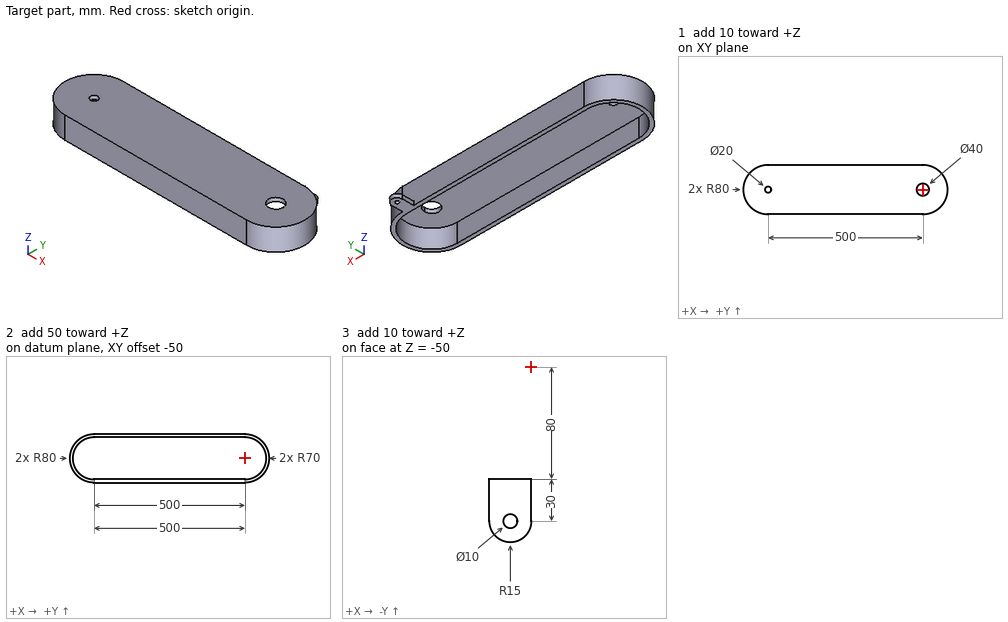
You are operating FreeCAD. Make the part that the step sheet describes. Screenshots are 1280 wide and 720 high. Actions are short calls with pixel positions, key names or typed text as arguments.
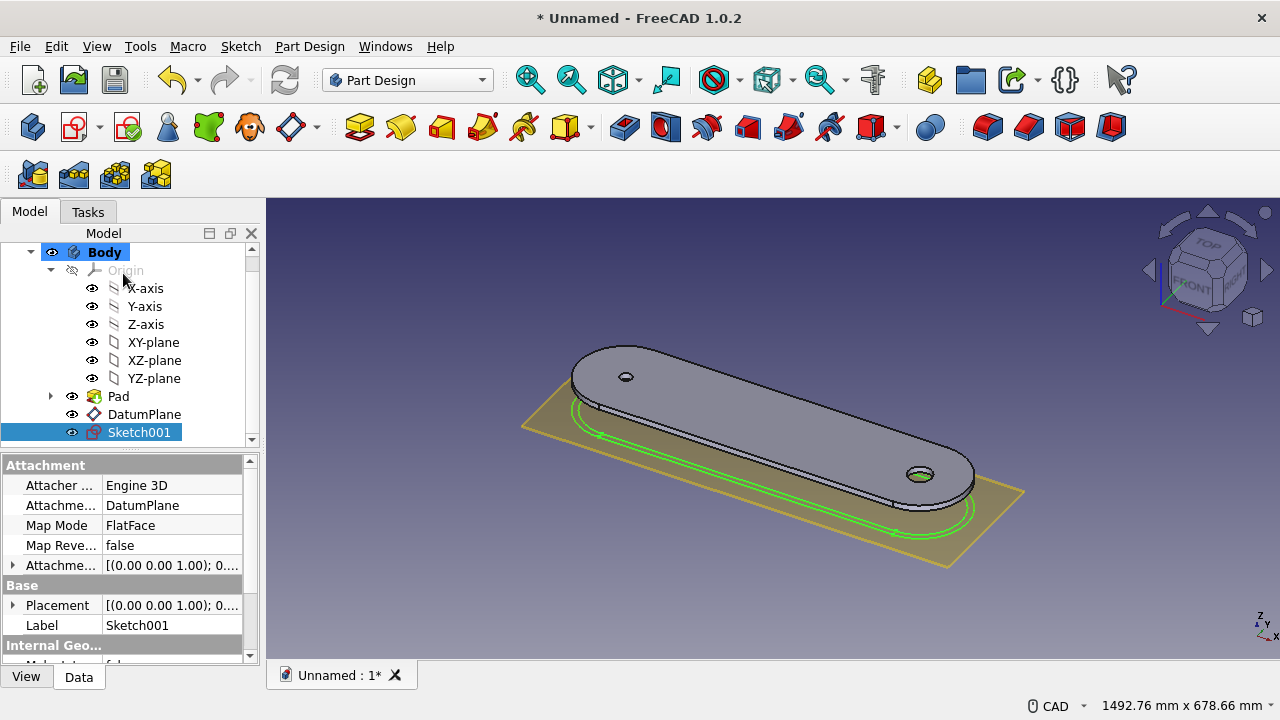
click(360, 128)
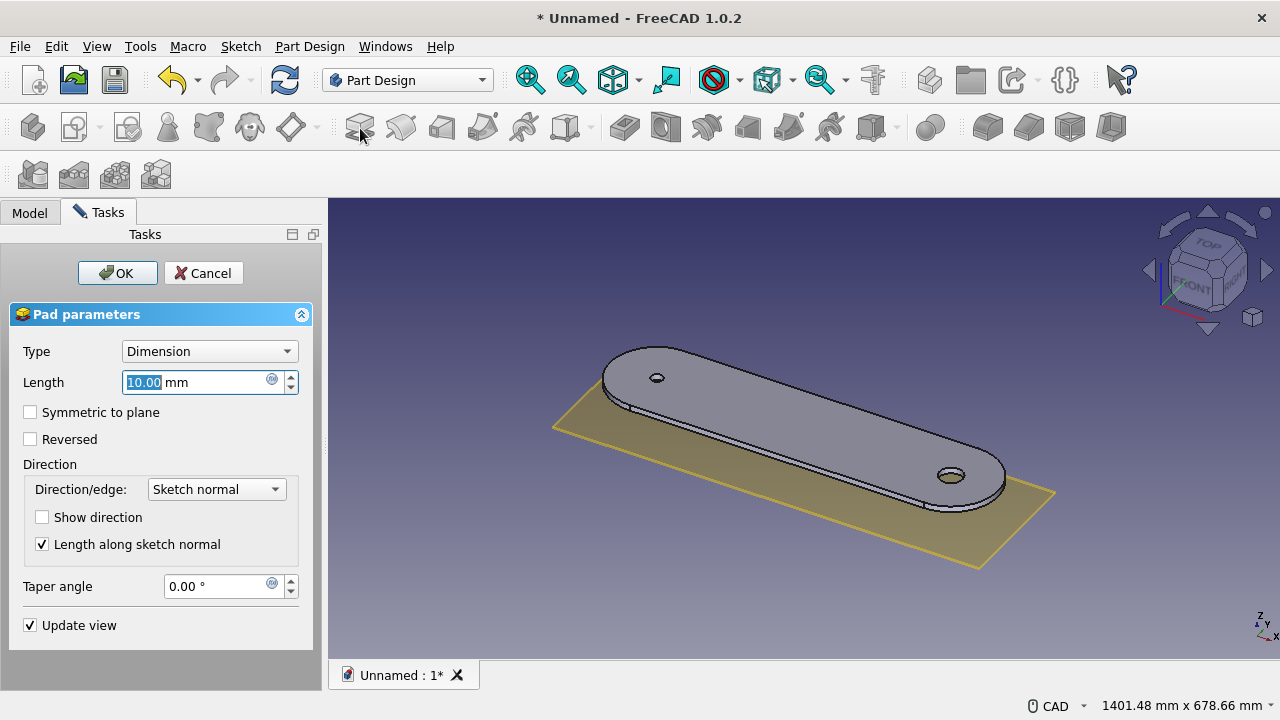
text(50)
key(Tab)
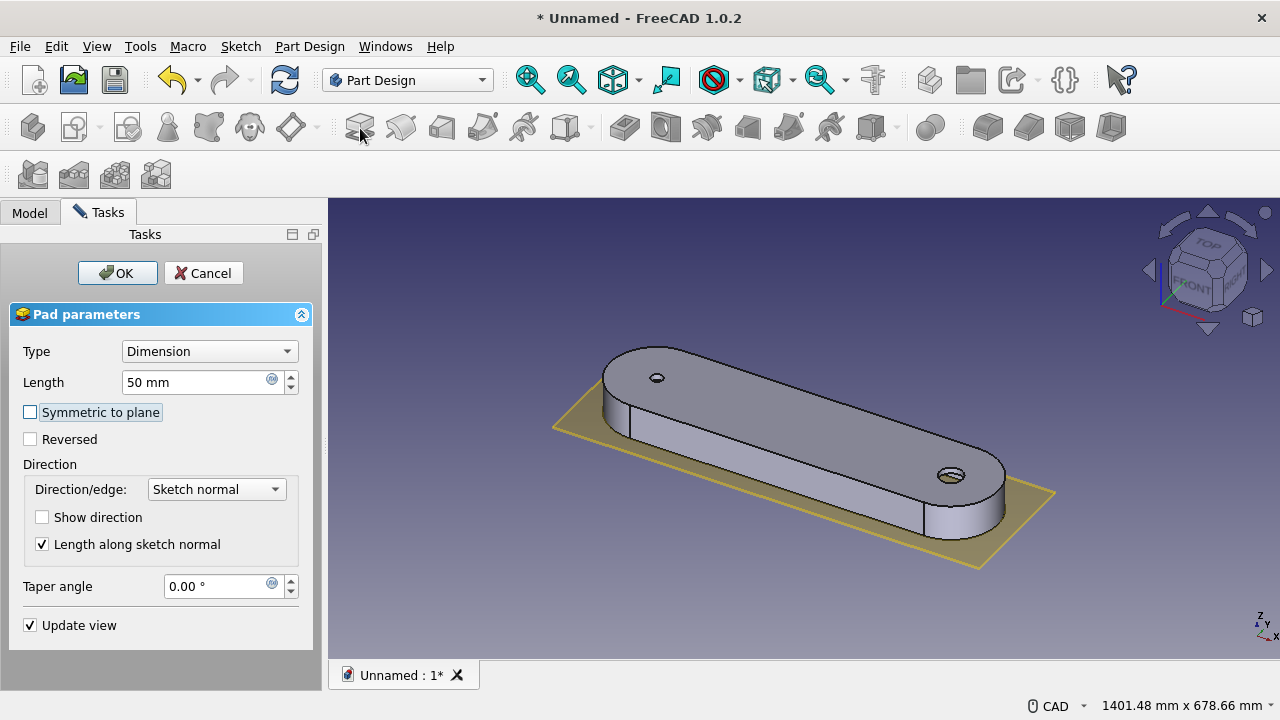
click(118, 273)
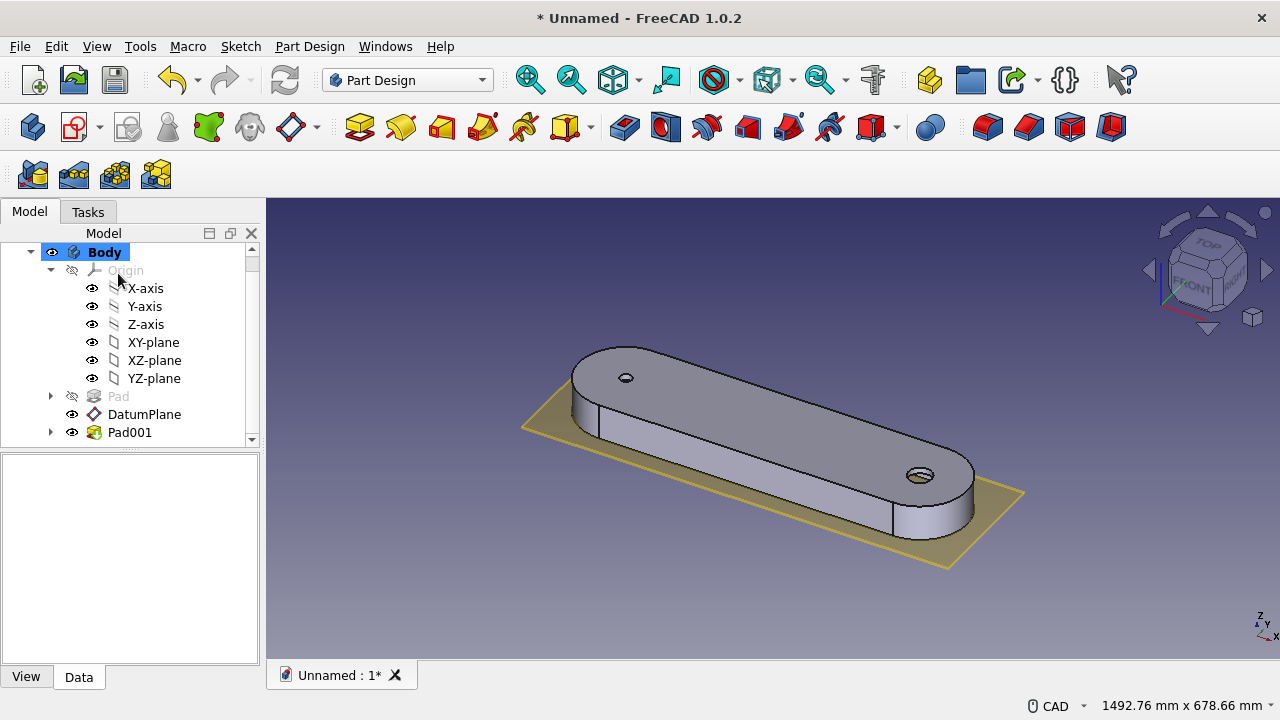
click(117, 414)
key(space)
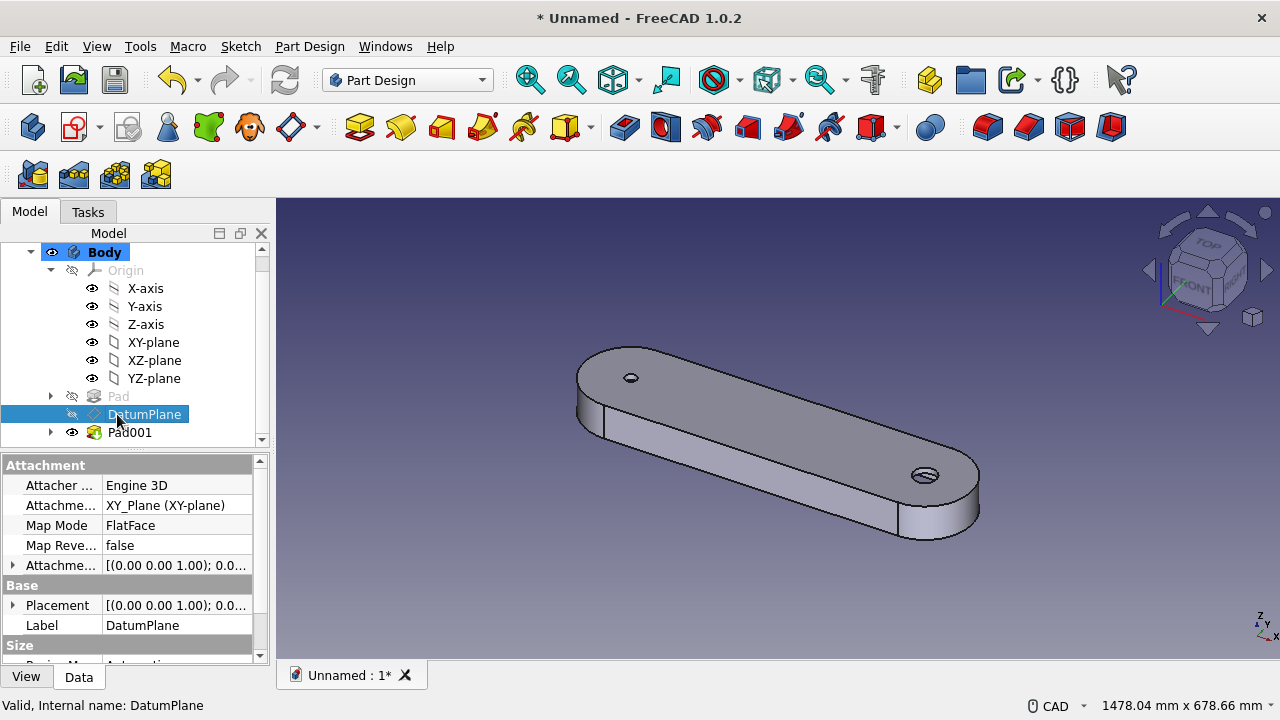
key(5)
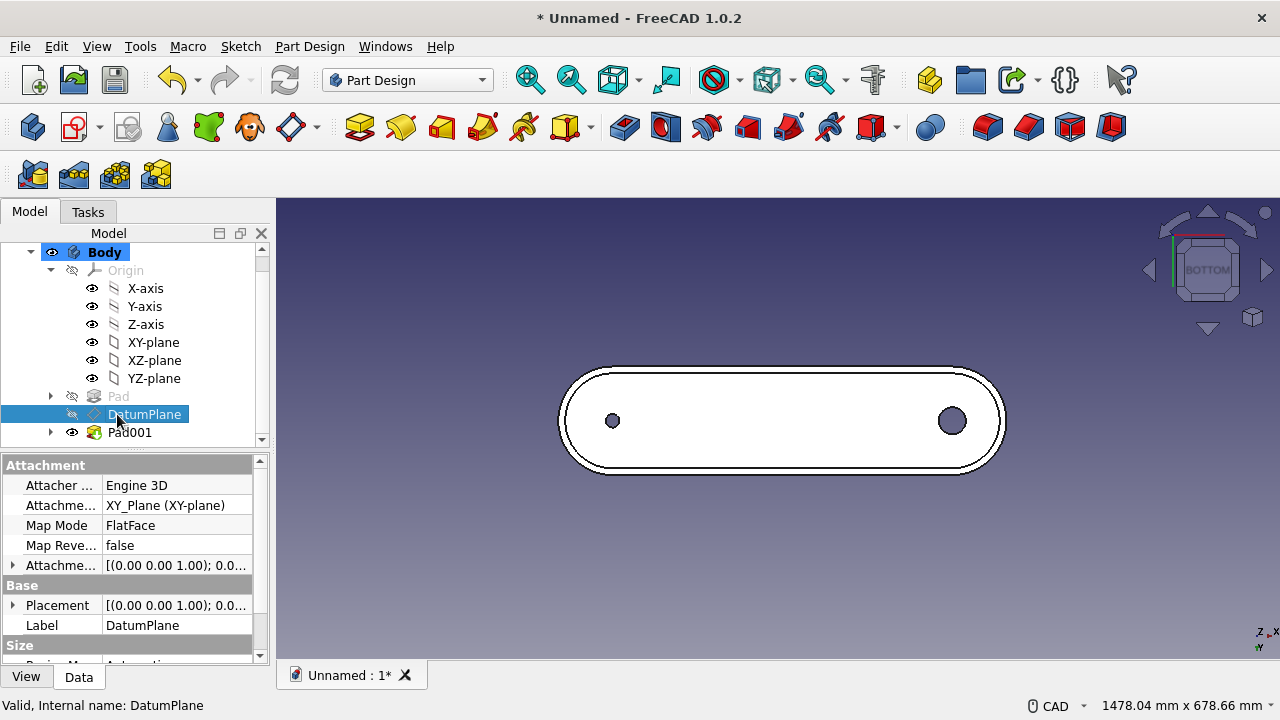
click(531, 80)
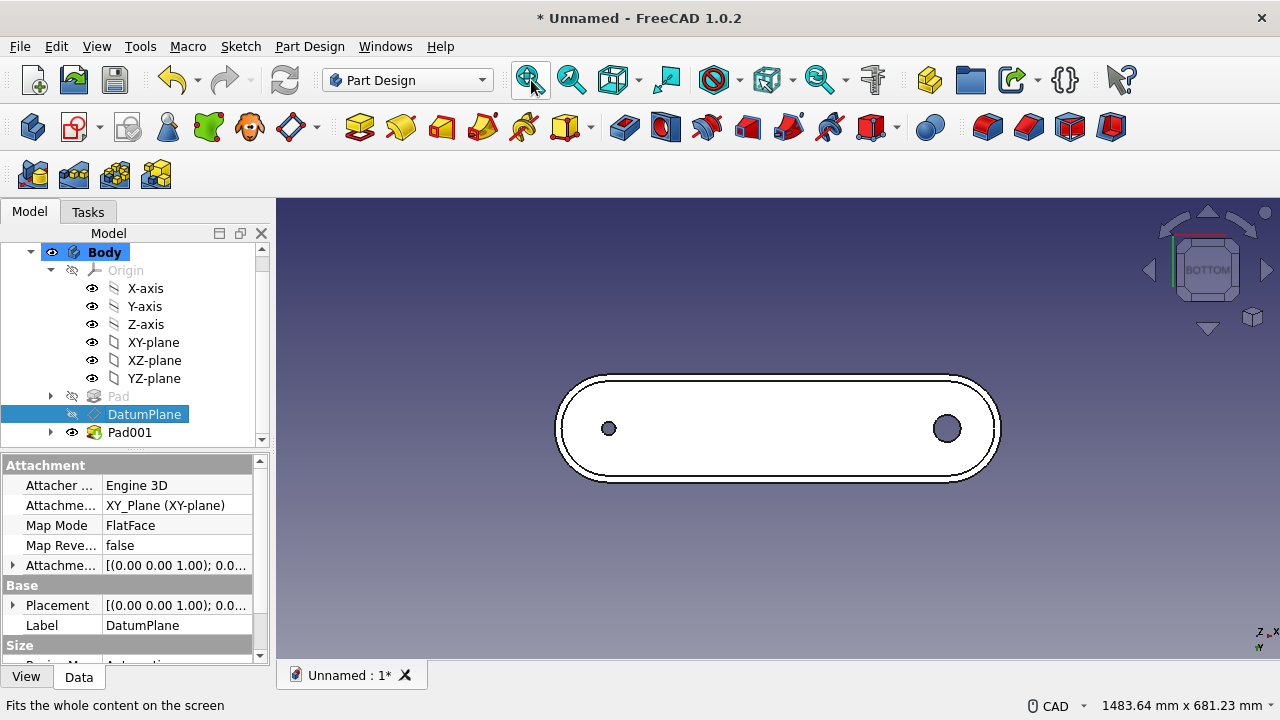
scroll(969, 381, up, 8)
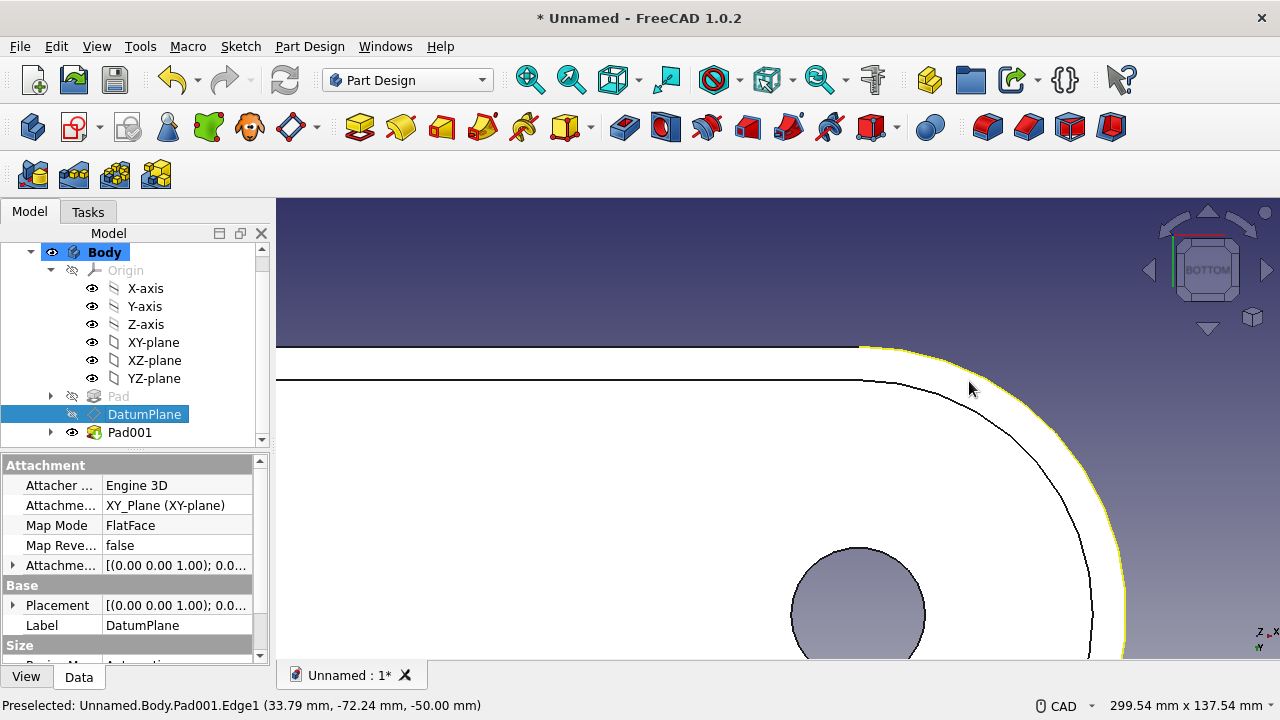
click(968, 384)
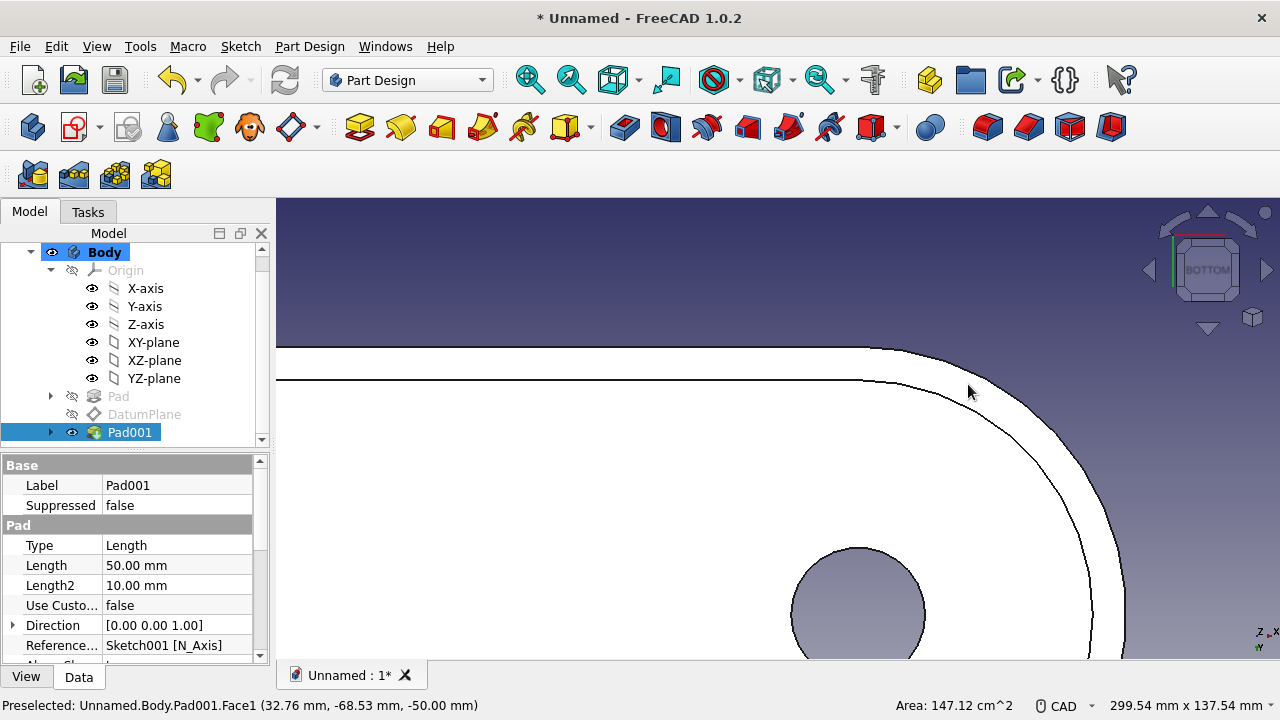
click(74, 128)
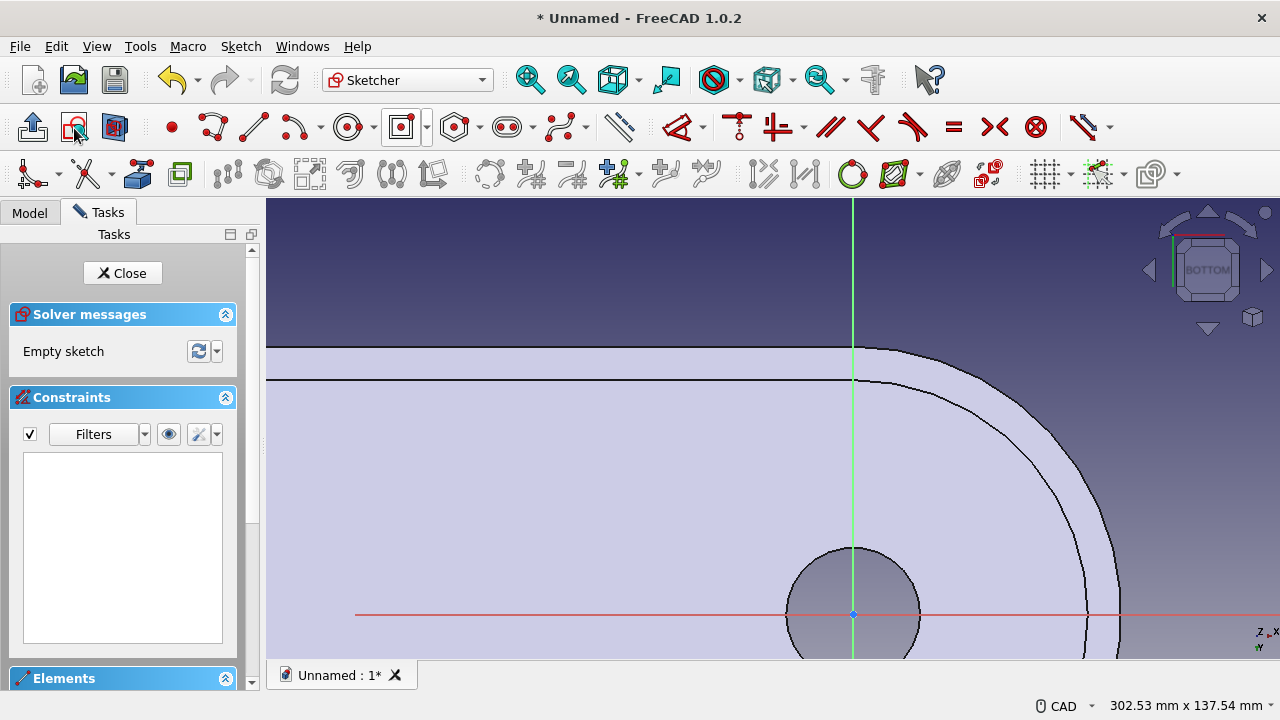
scroll(704, 428, down, 5)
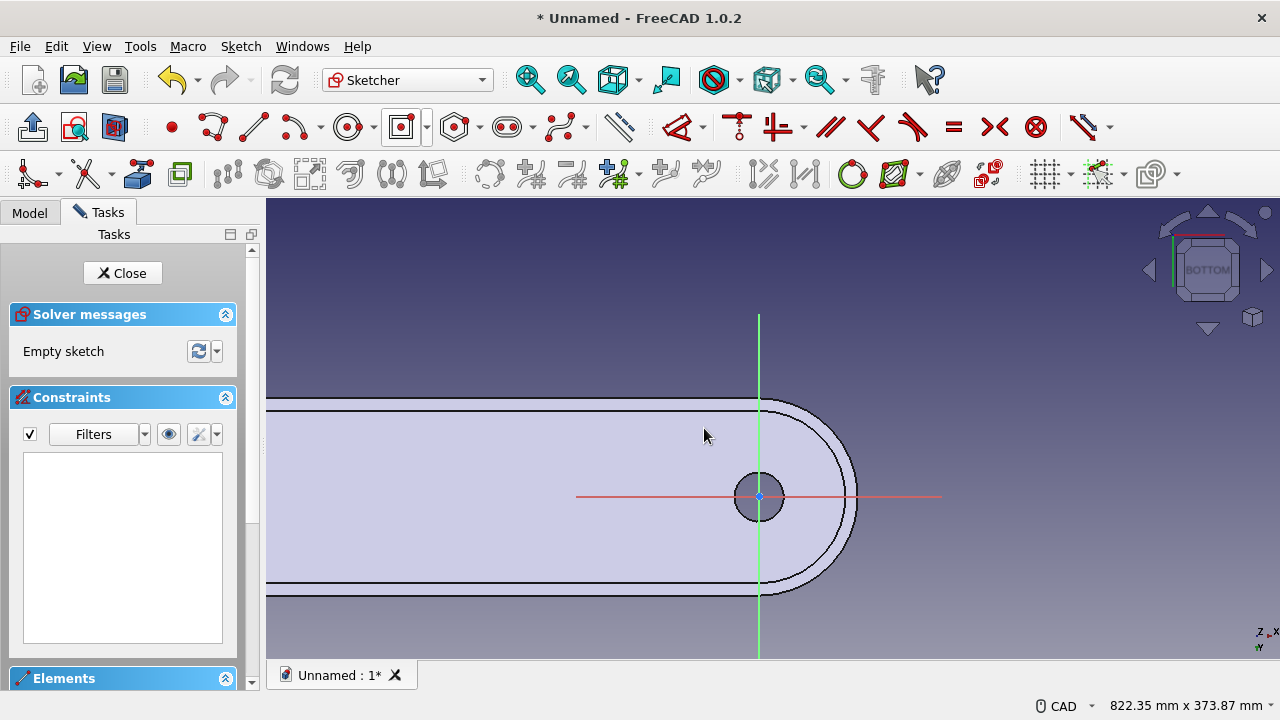
scroll(704, 428, down, 5)